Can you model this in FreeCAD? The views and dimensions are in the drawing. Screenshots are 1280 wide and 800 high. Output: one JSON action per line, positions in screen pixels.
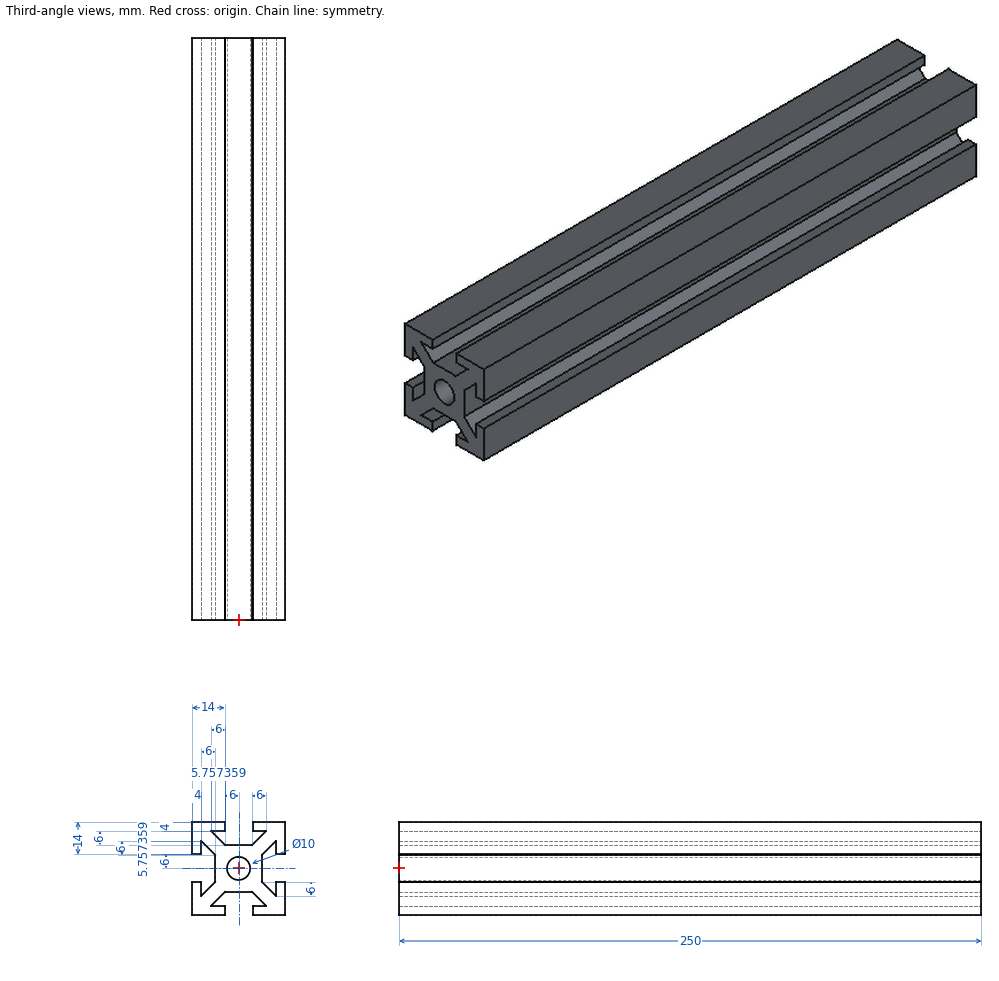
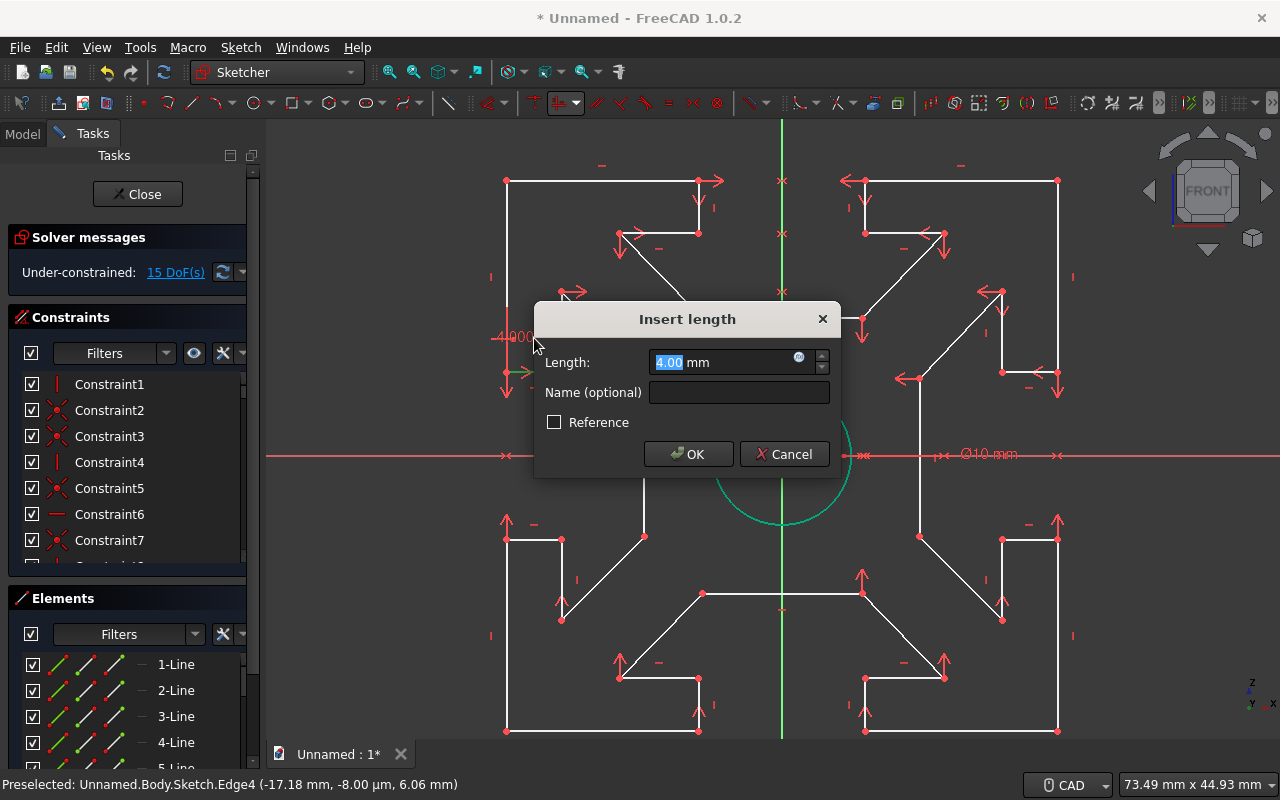
{"action": "type", "text": "4"}
{"action": "key", "text": "Return"}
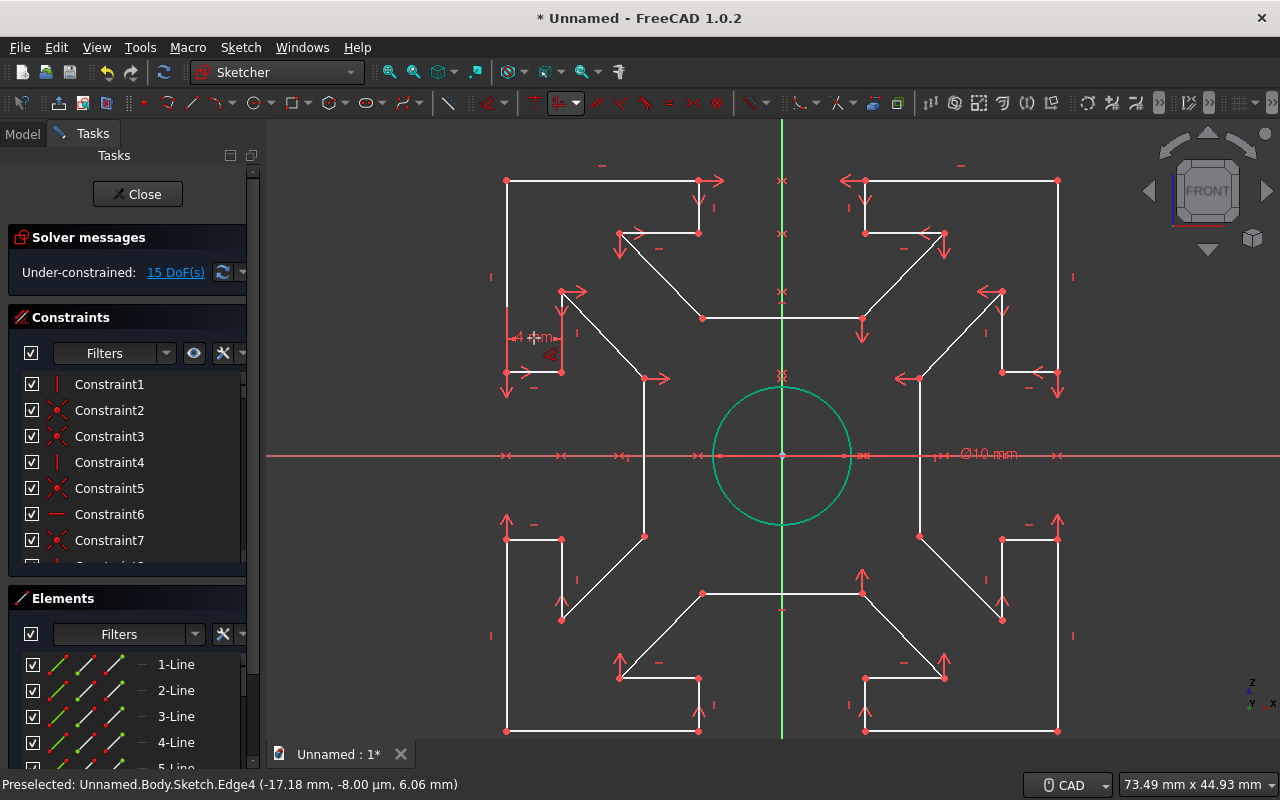
{"action": "left_click", "coordinate": [699, 197]}
{"action": "left_click", "coordinate": [665, 207]}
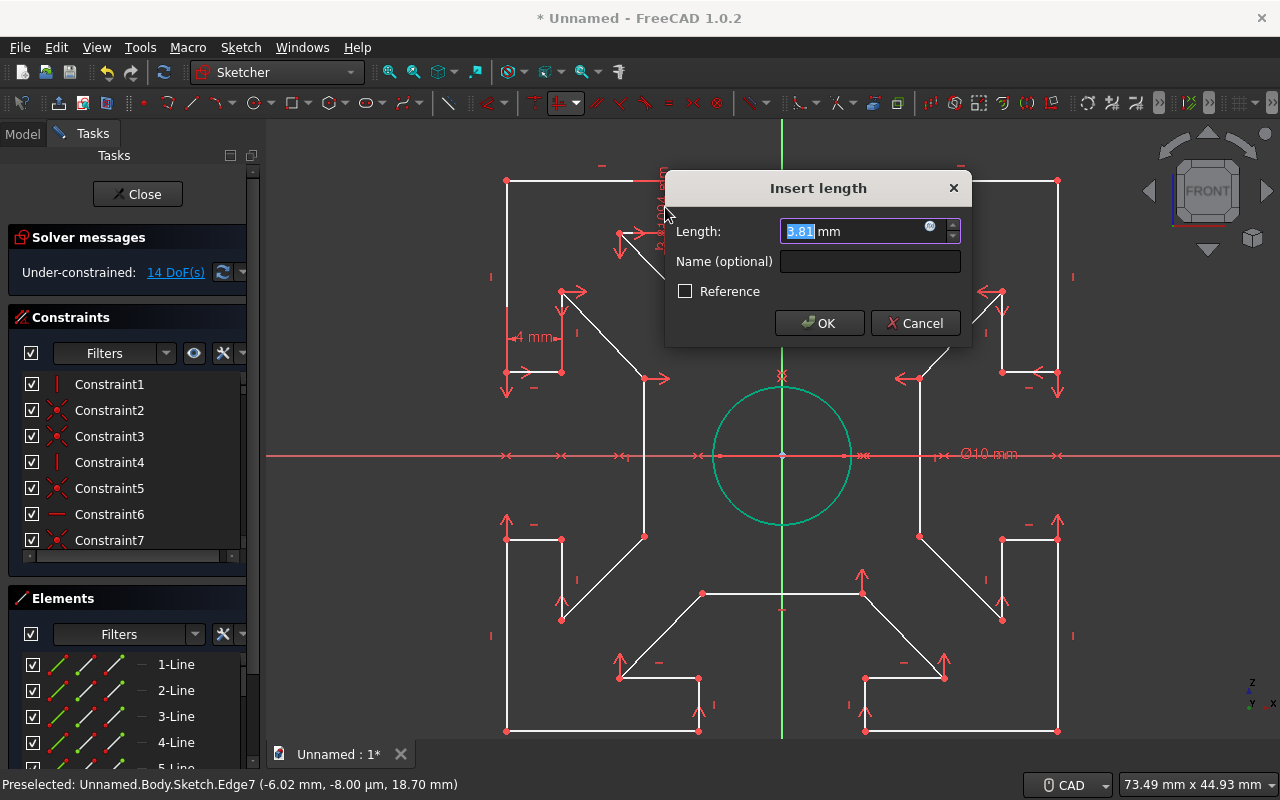
{"action": "type", "text": "4"}
{"action": "key", "text": "Return"}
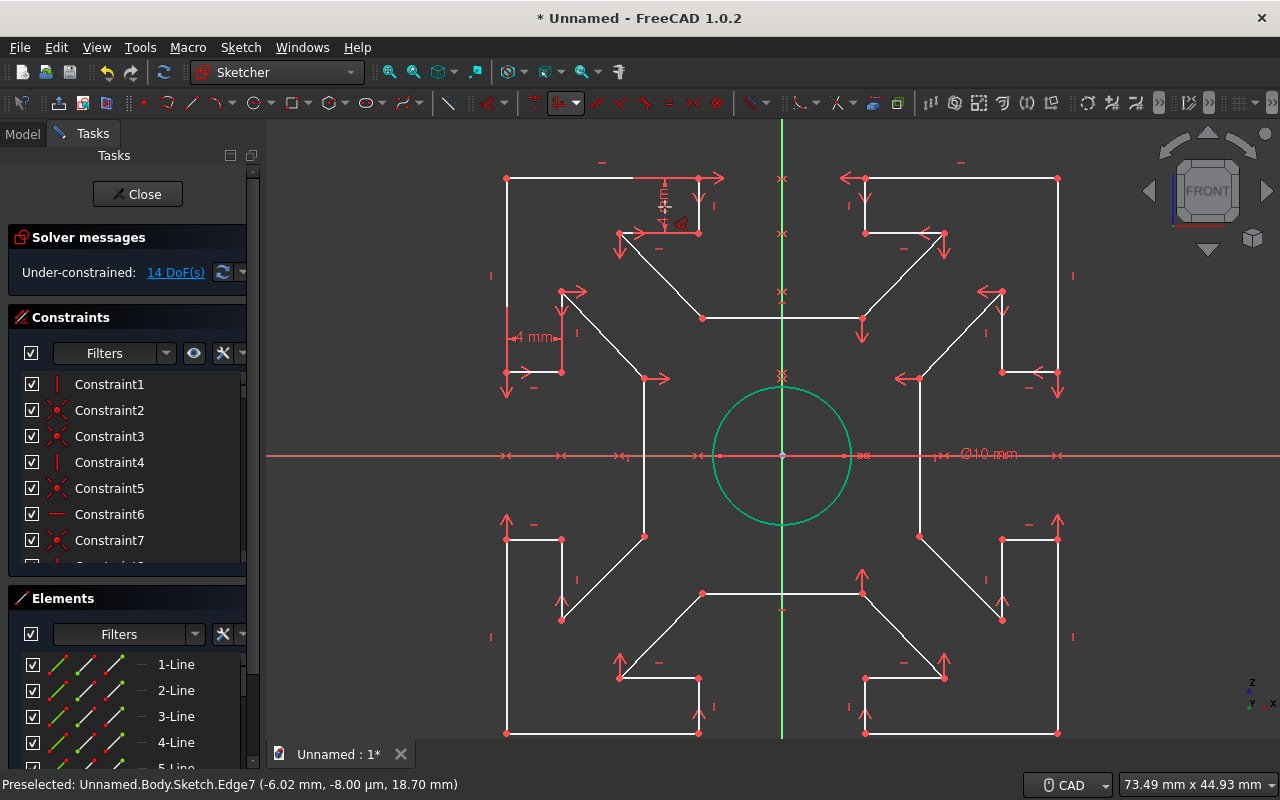
{"action": "left_click", "coordinate": [507, 314]}
{"action": "left_click", "coordinate": [473, 275]}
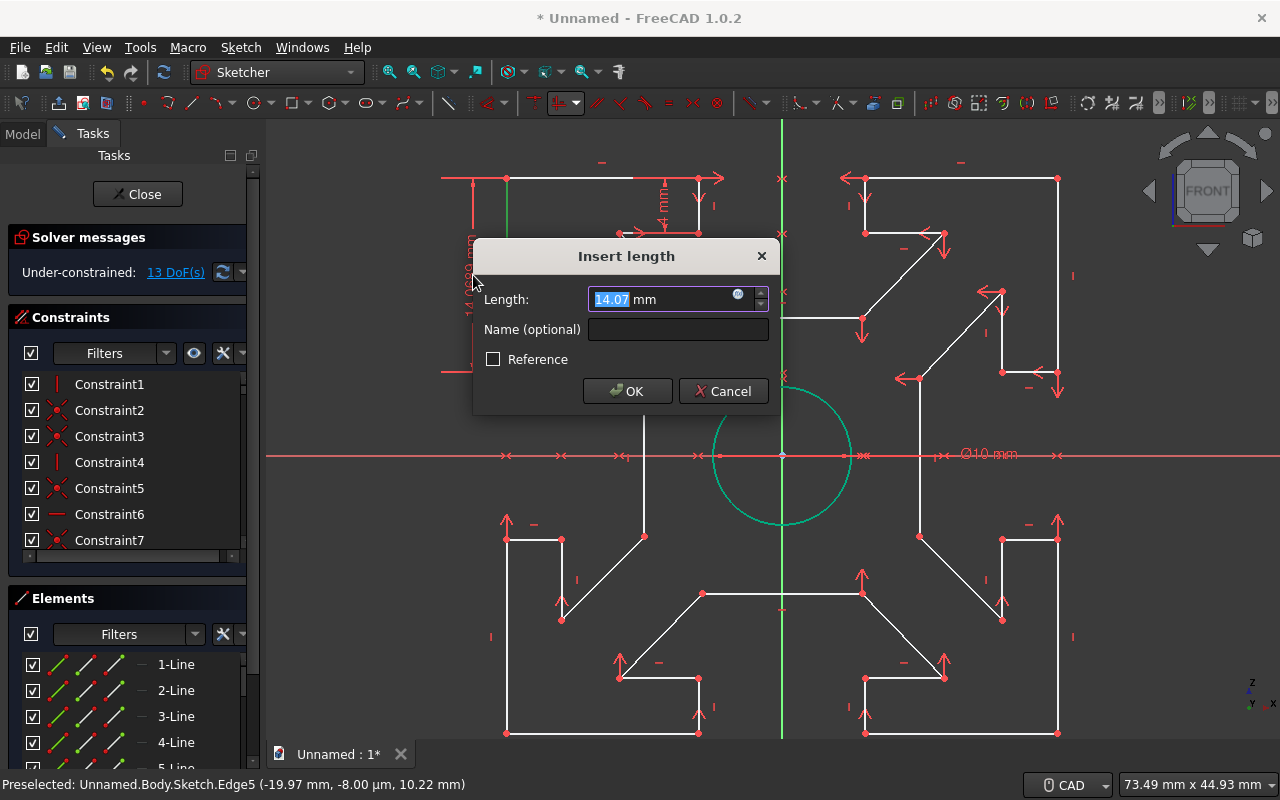
{"action": "type", "text": "14"}
{"action": "key", "text": "Return"}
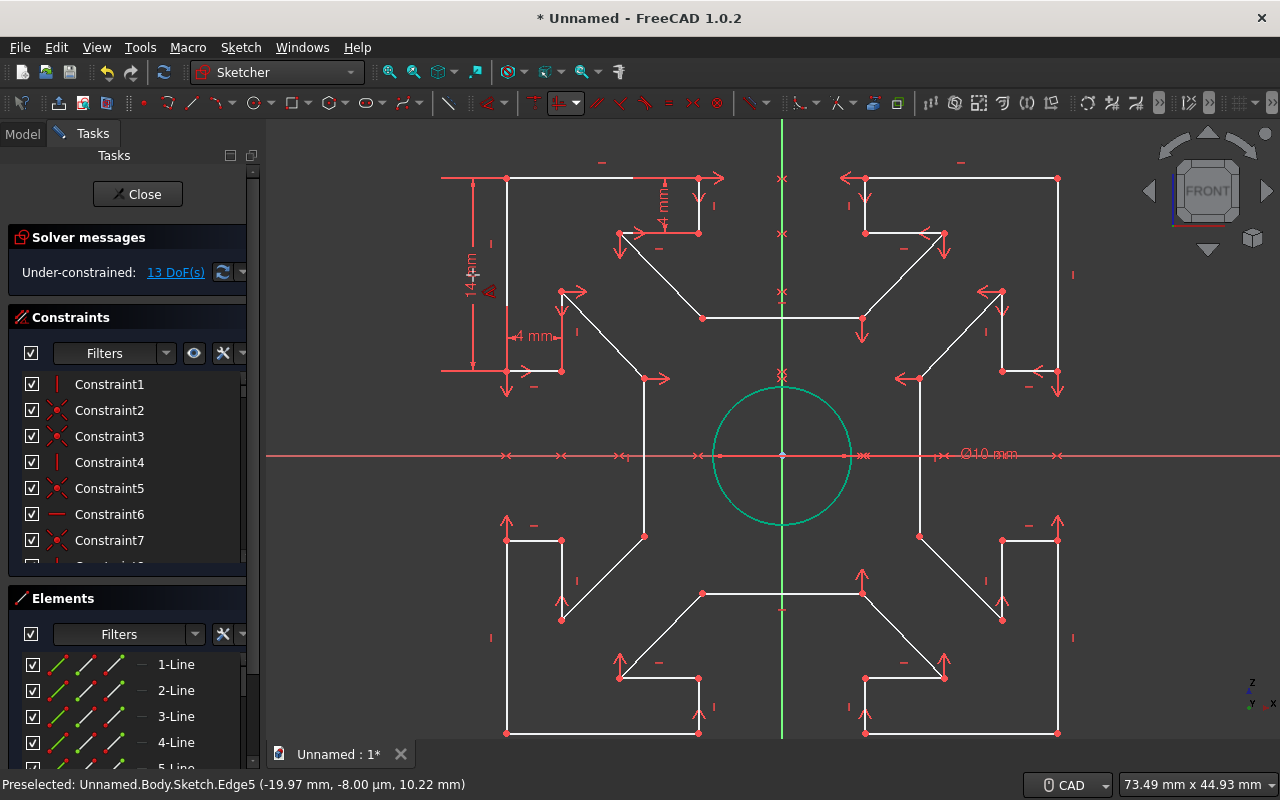
{"action": "left_click", "coordinate": [564, 178]}
{"action": "left_click", "coordinate": [559, 212]}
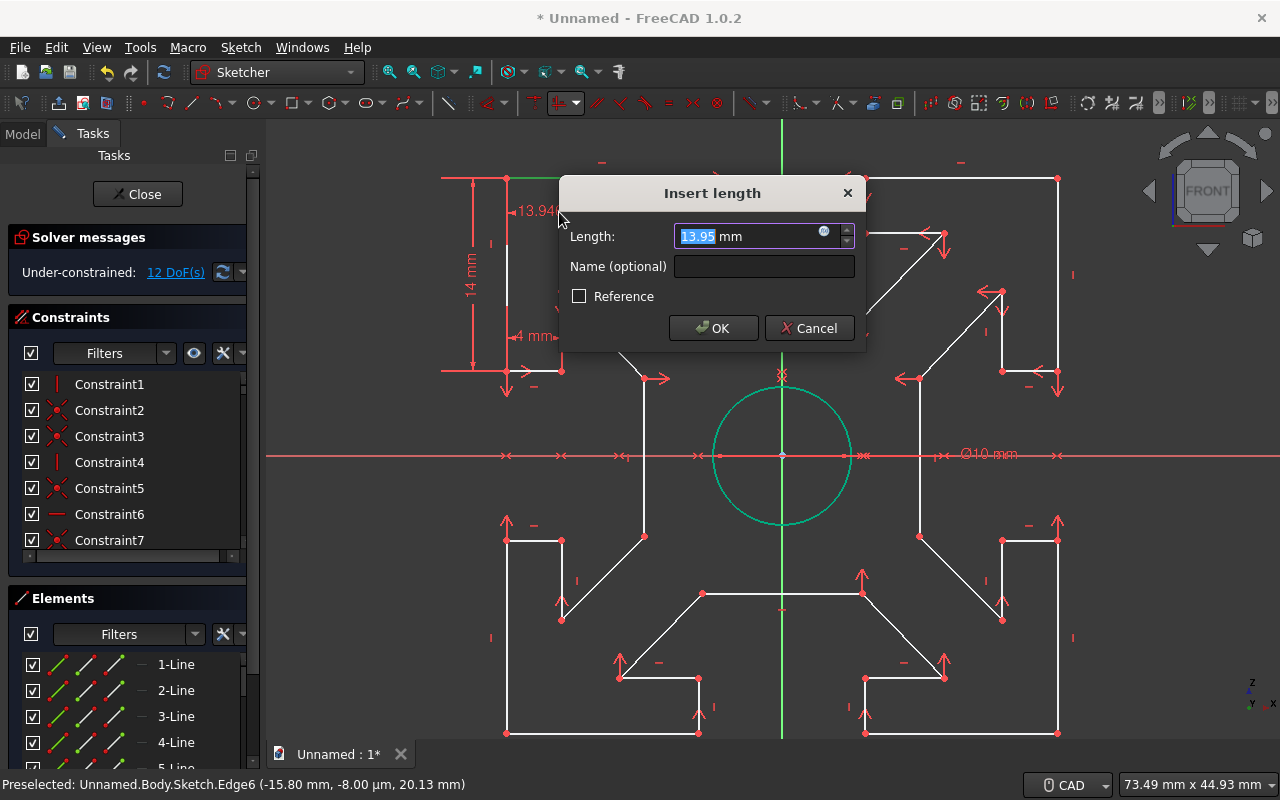
{"action": "type", "text": "14"}
{"action": "key", "text": "Return"}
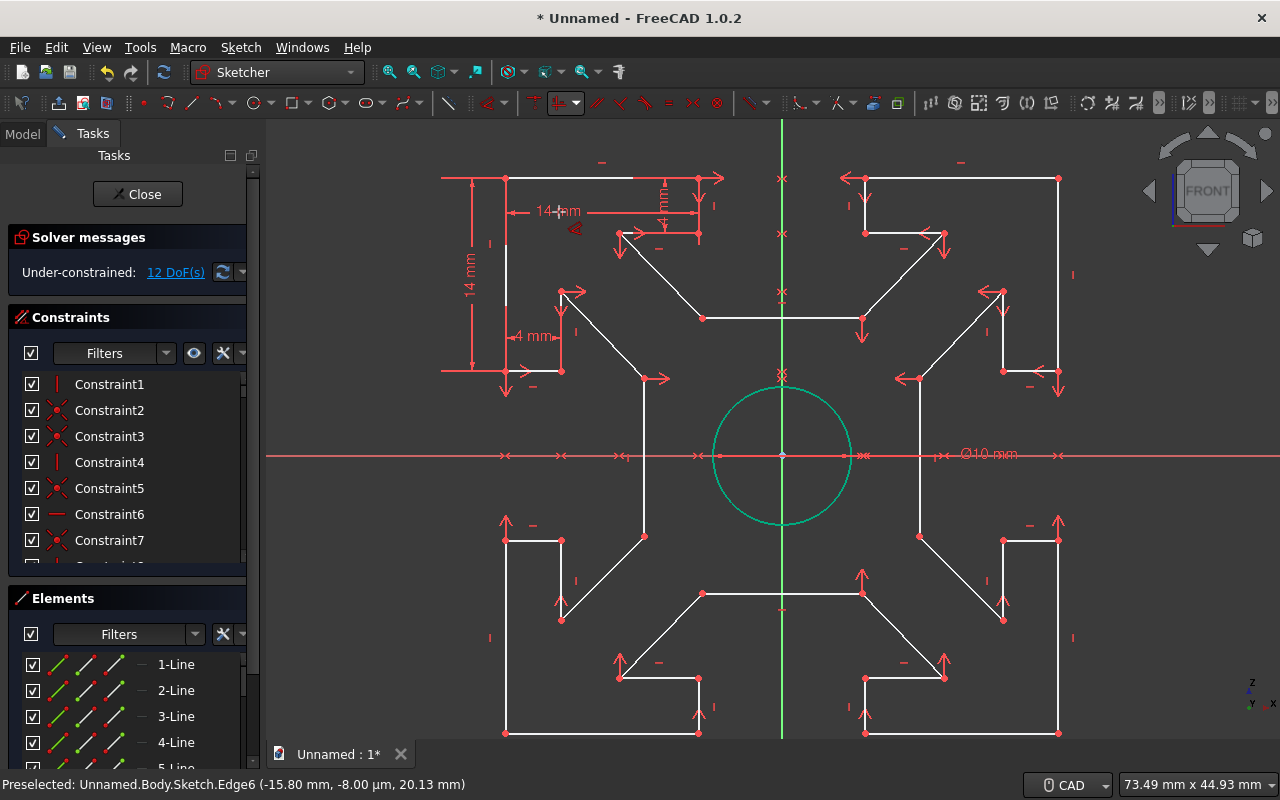
{"action": "left_click", "coordinate": [561, 371]}
{"action": "left_click", "coordinate": [527, 414]}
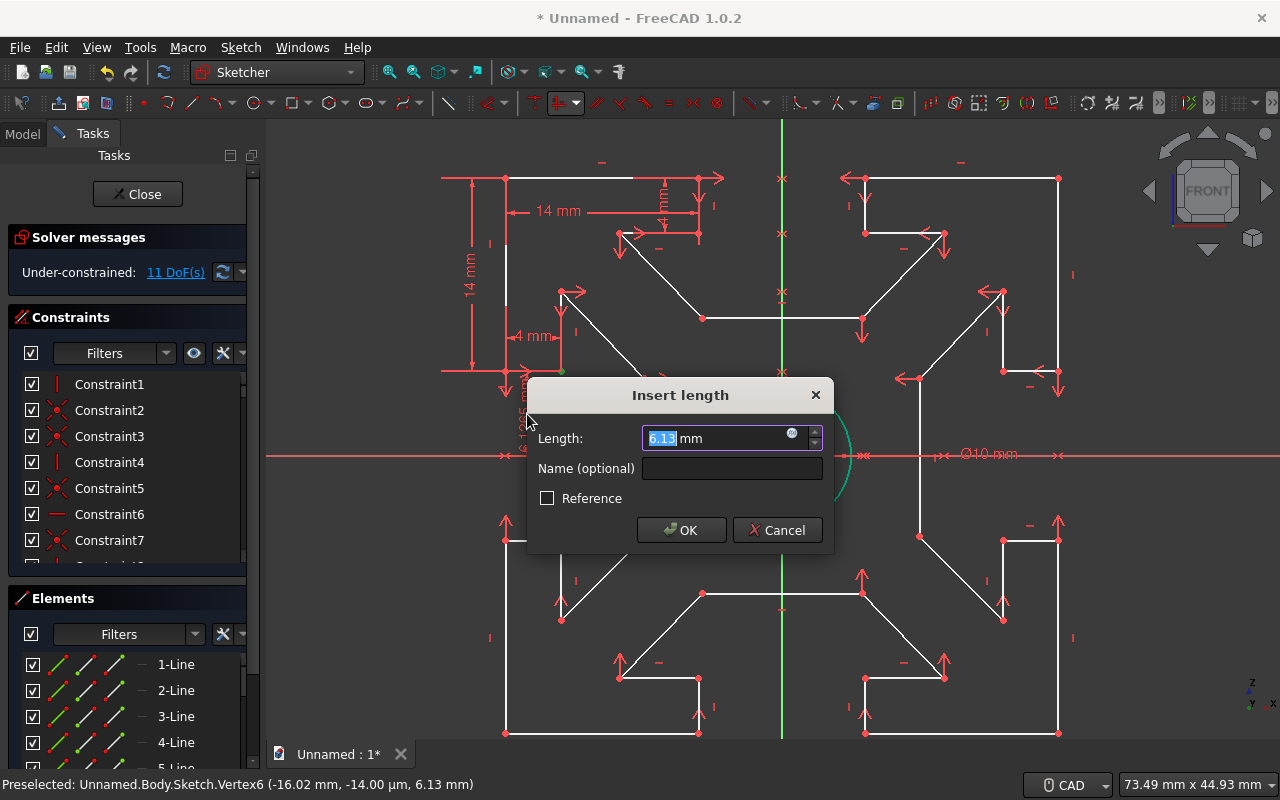
{"action": "type", "text": "6"}
{"action": "key", "text": "Return"}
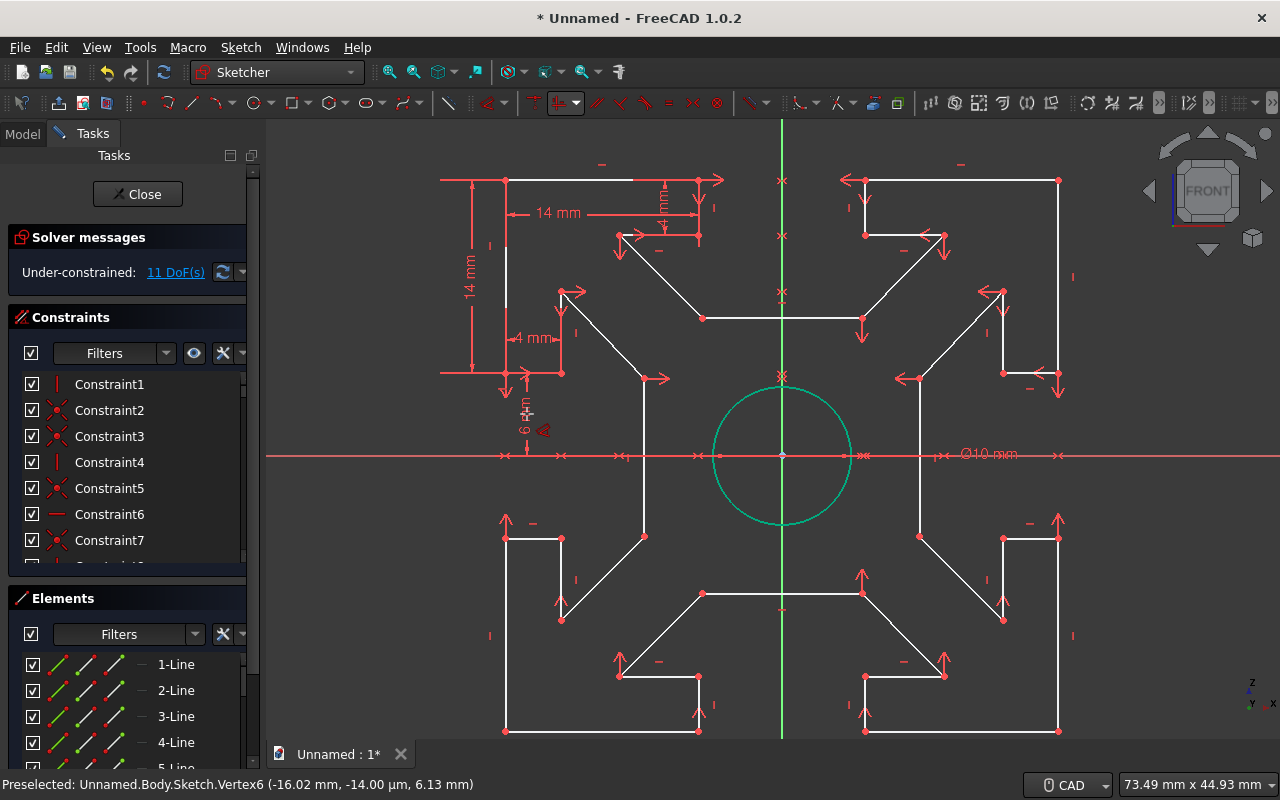
{"action": "left_click", "coordinate": [699, 180]}
{"action": "left_click", "coordinate": [741, 490]}